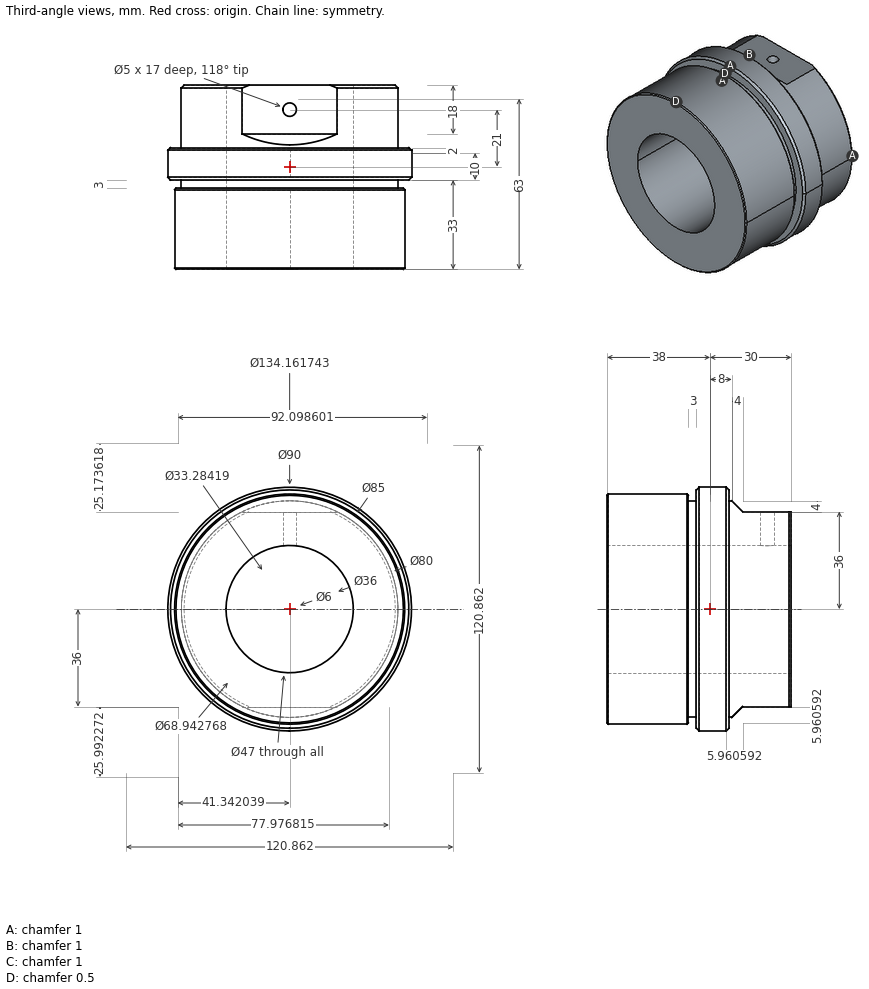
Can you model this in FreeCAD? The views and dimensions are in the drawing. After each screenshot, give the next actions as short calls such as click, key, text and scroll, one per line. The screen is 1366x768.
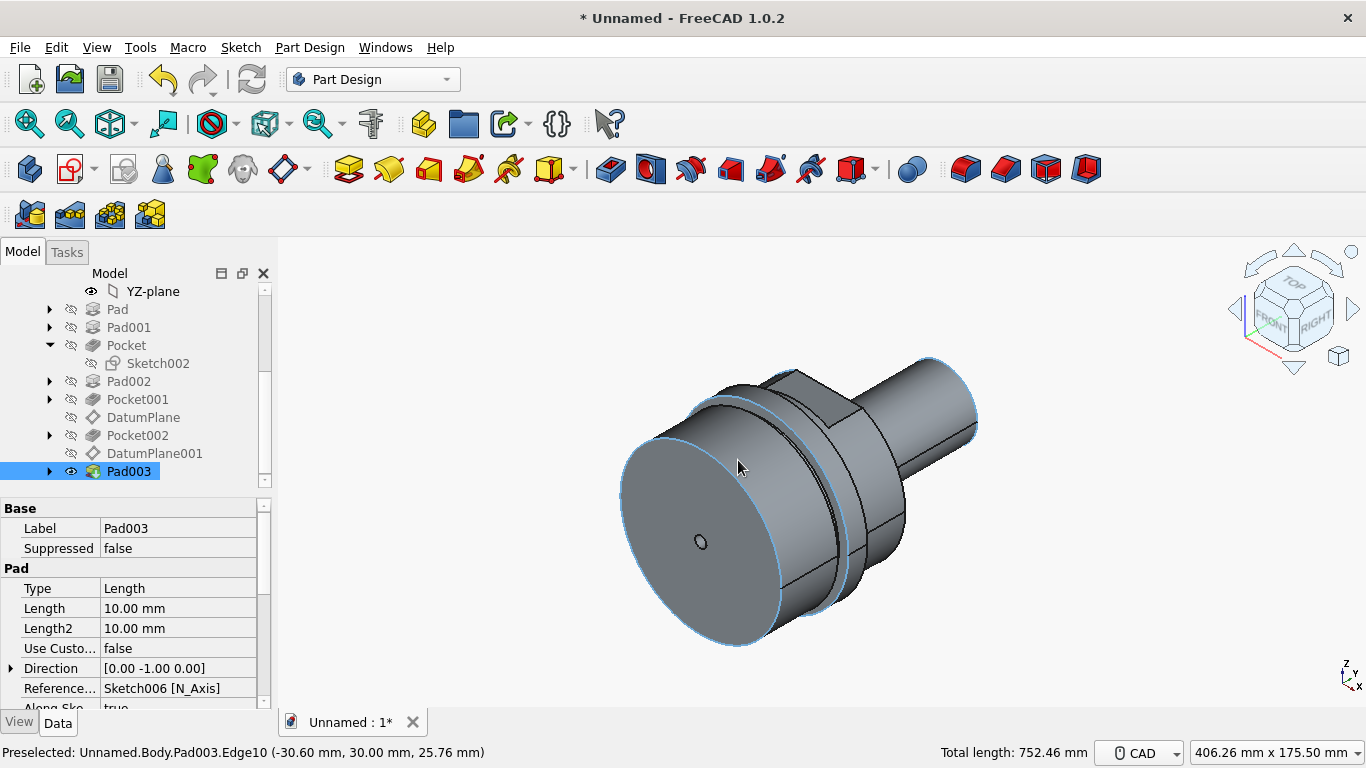
key(1)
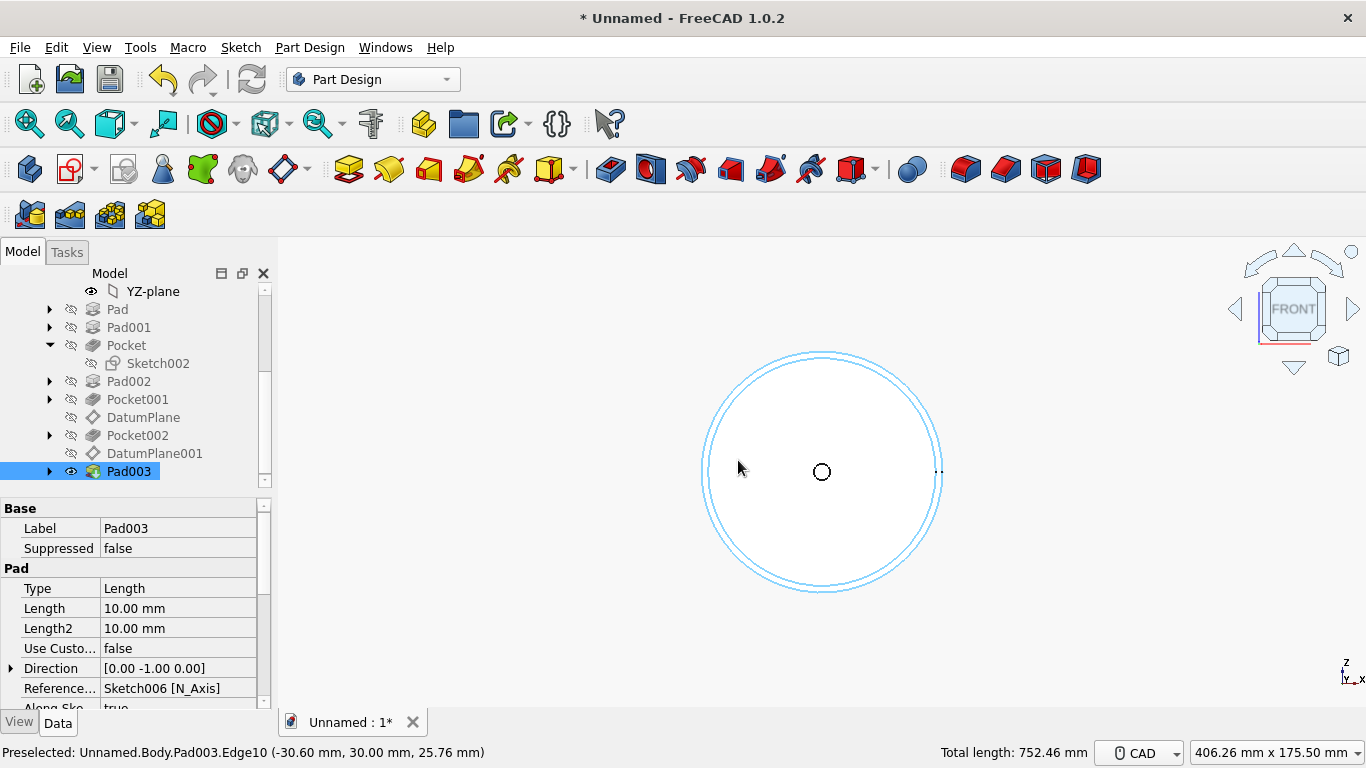
key(3)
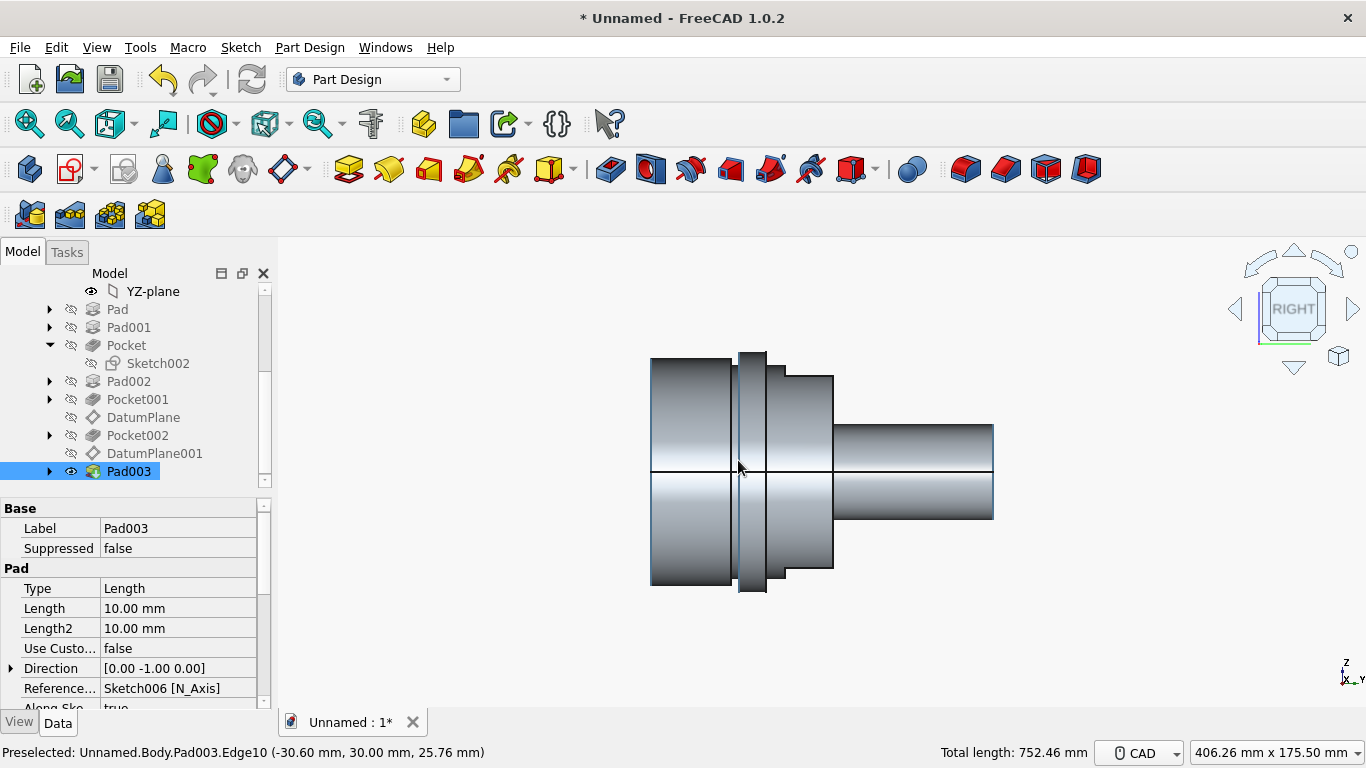
click(833, 517, ctrl)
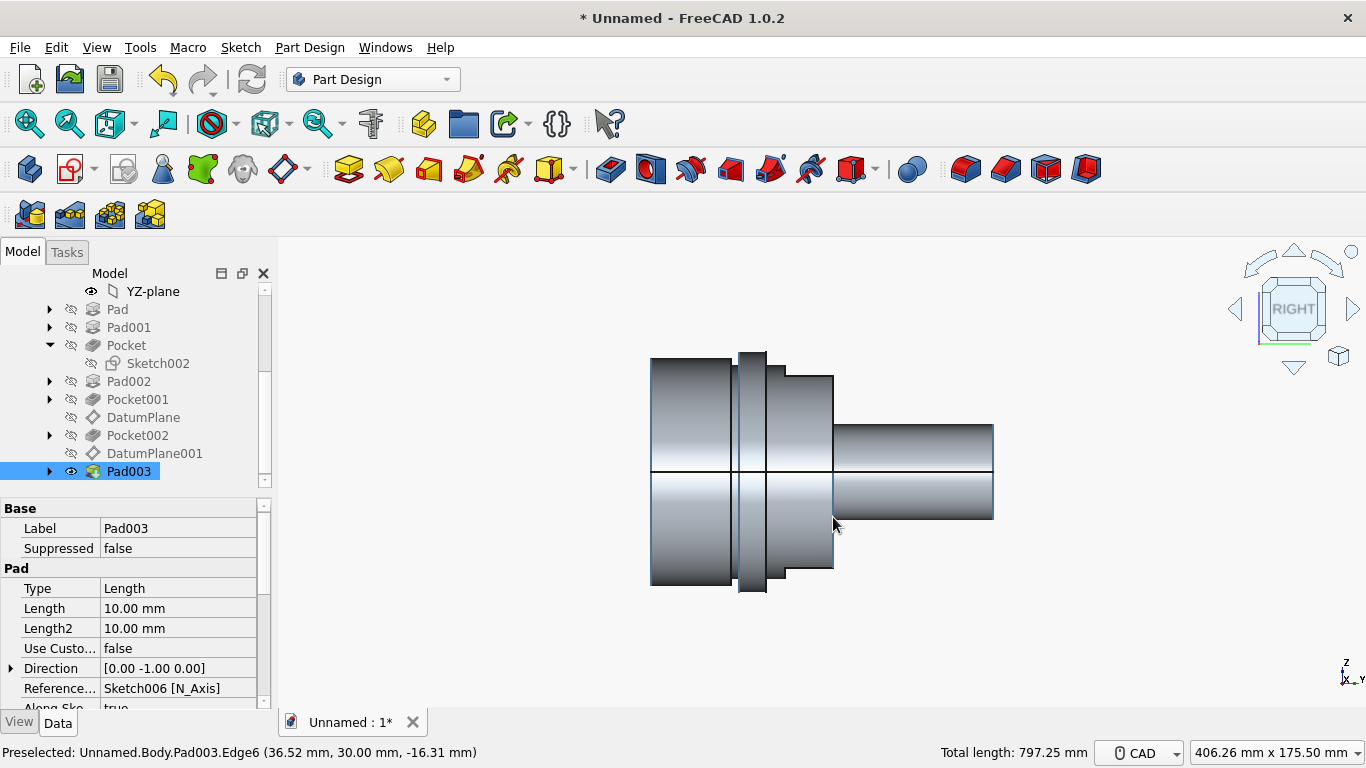
click(1006, 170)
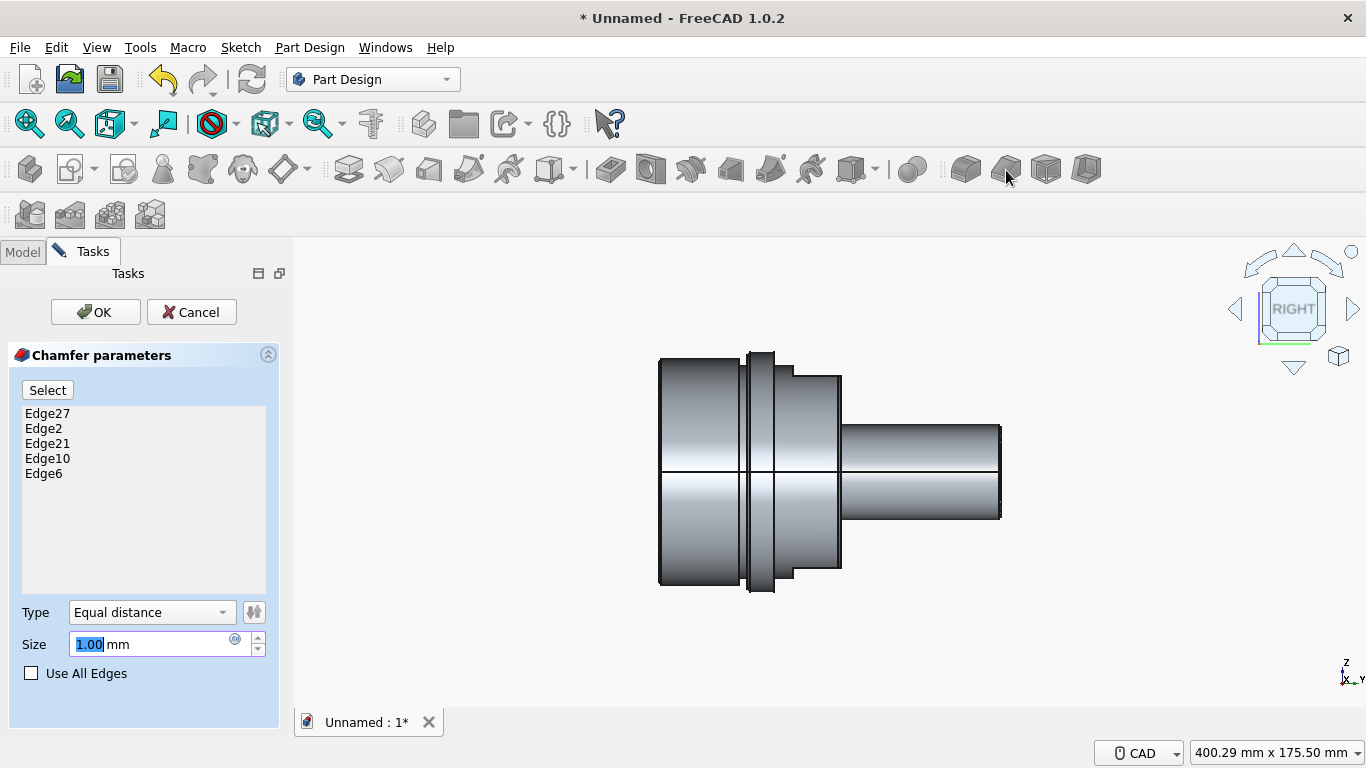
text(1)
key(Tab)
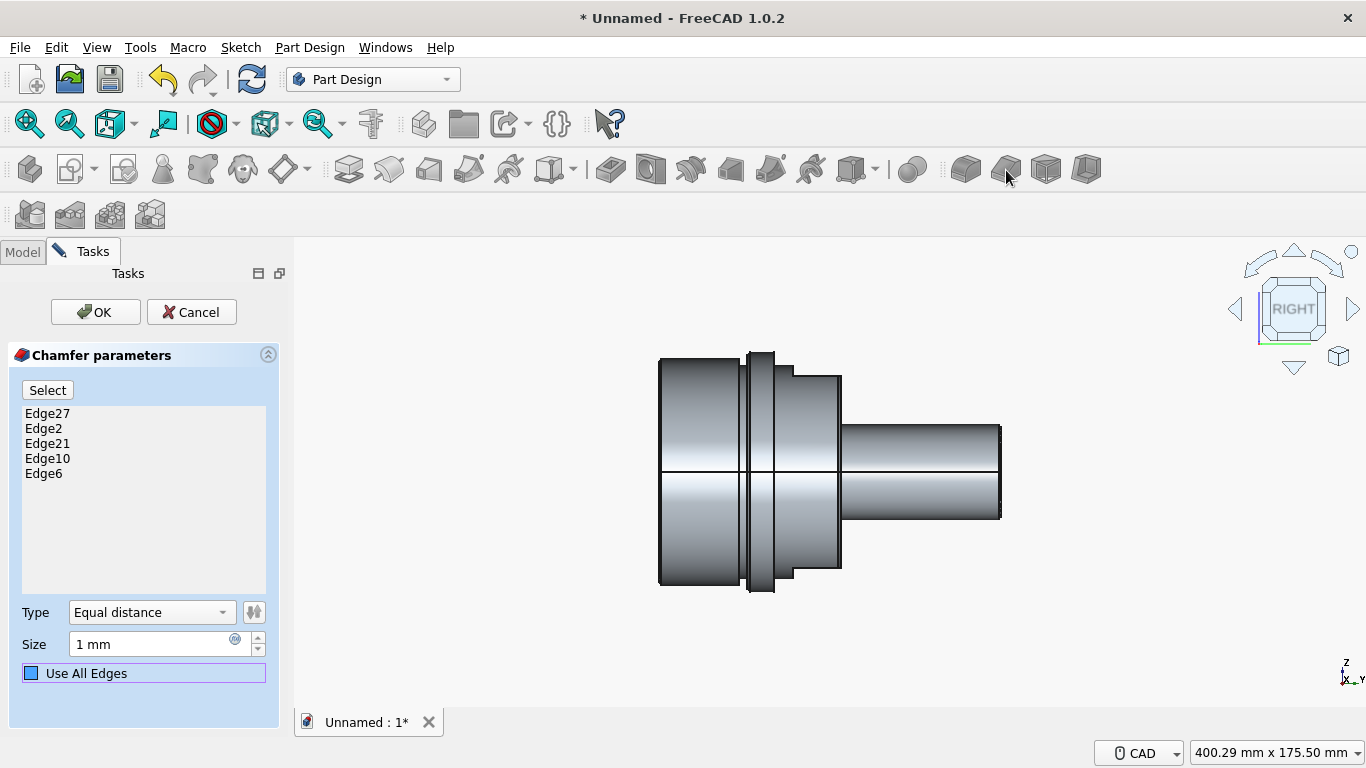
click(96, 312)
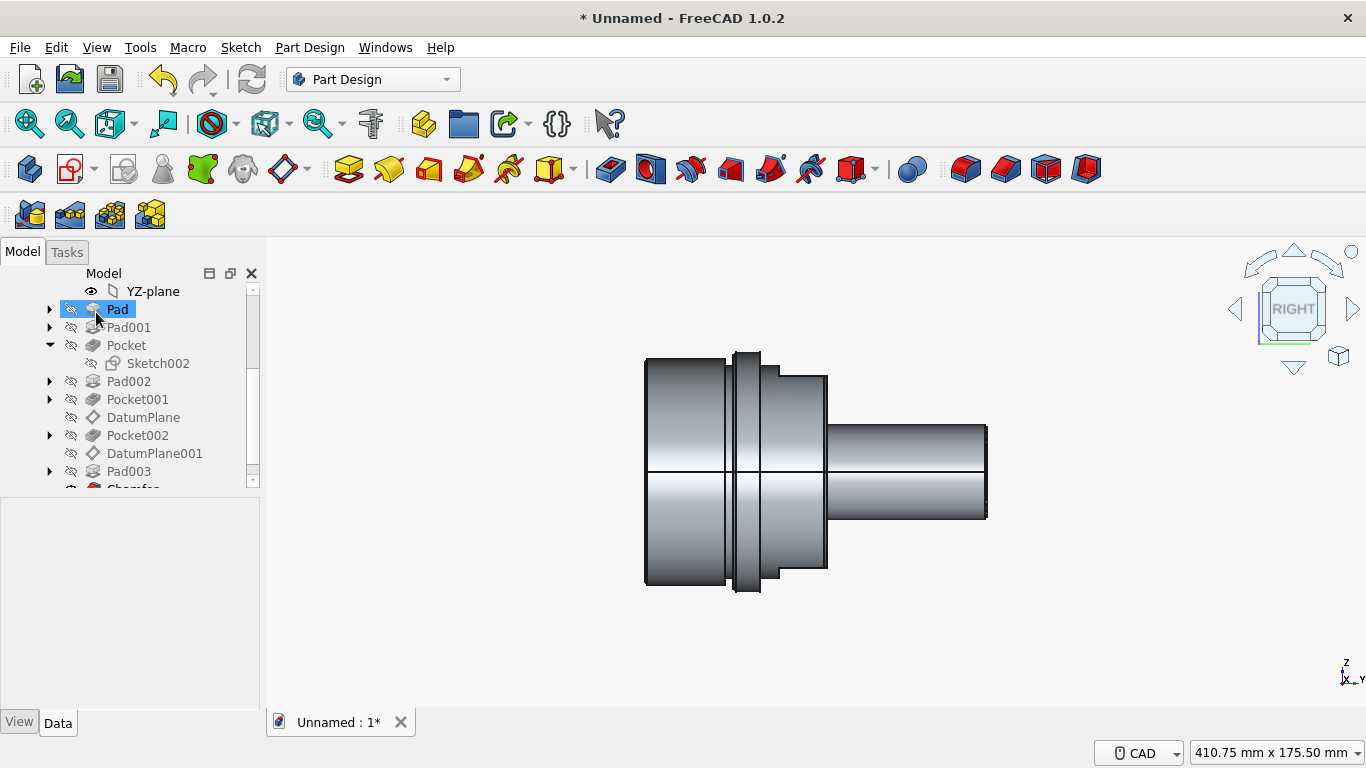
click(70, 170)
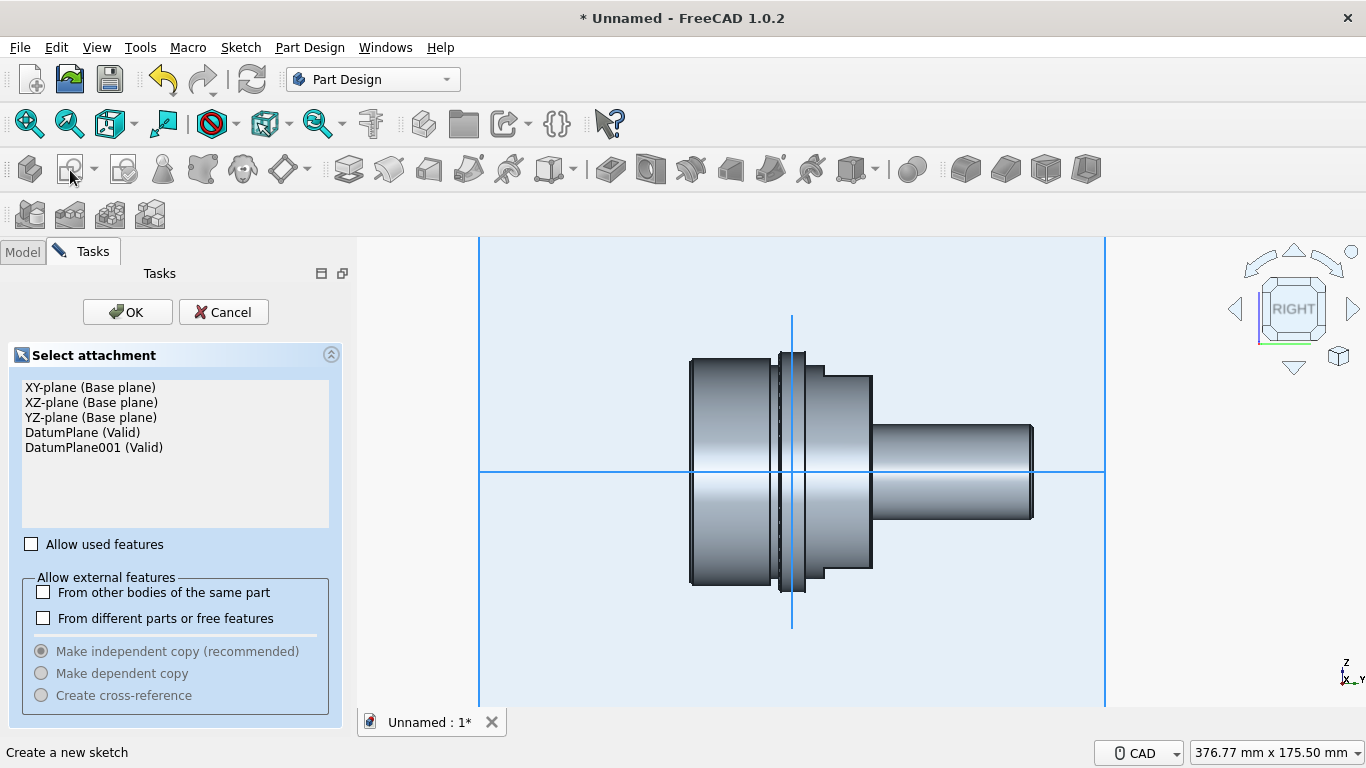
click(82, 418)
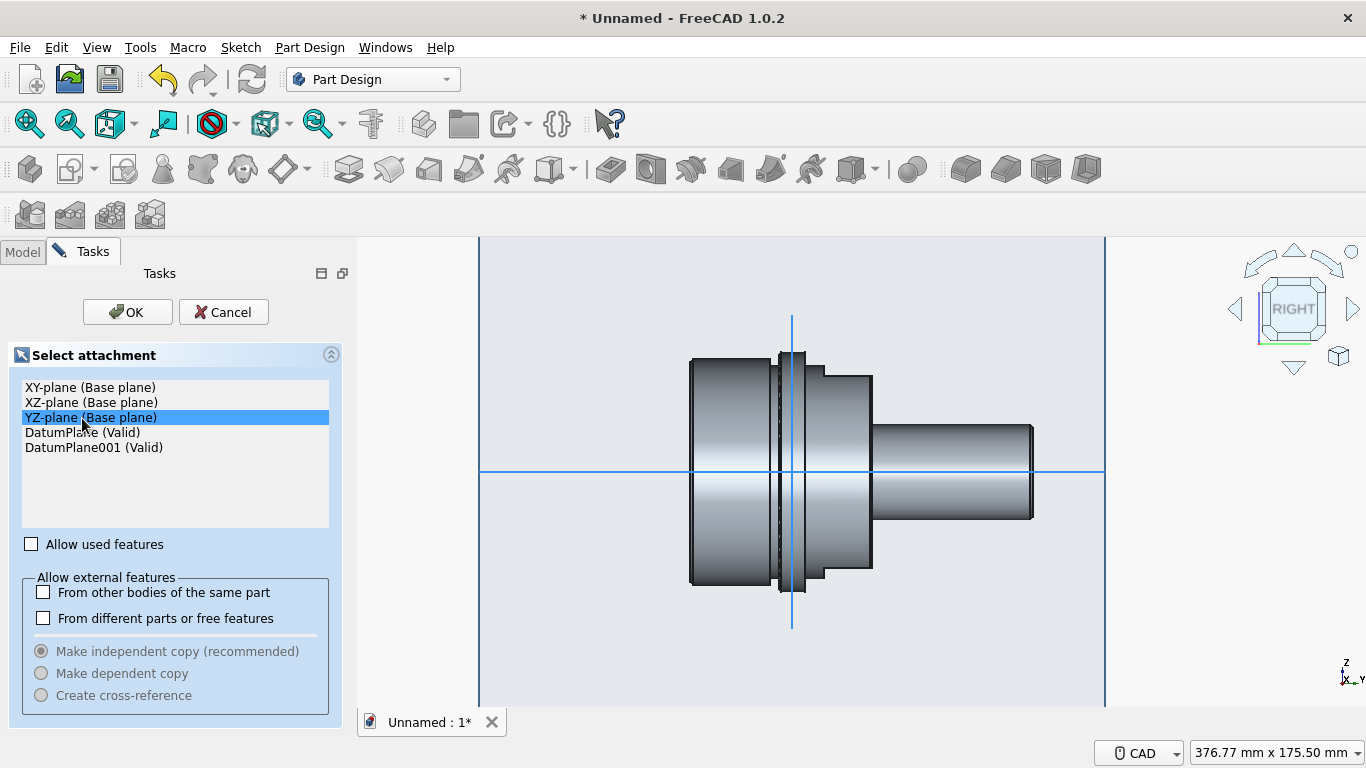
click(128, 312)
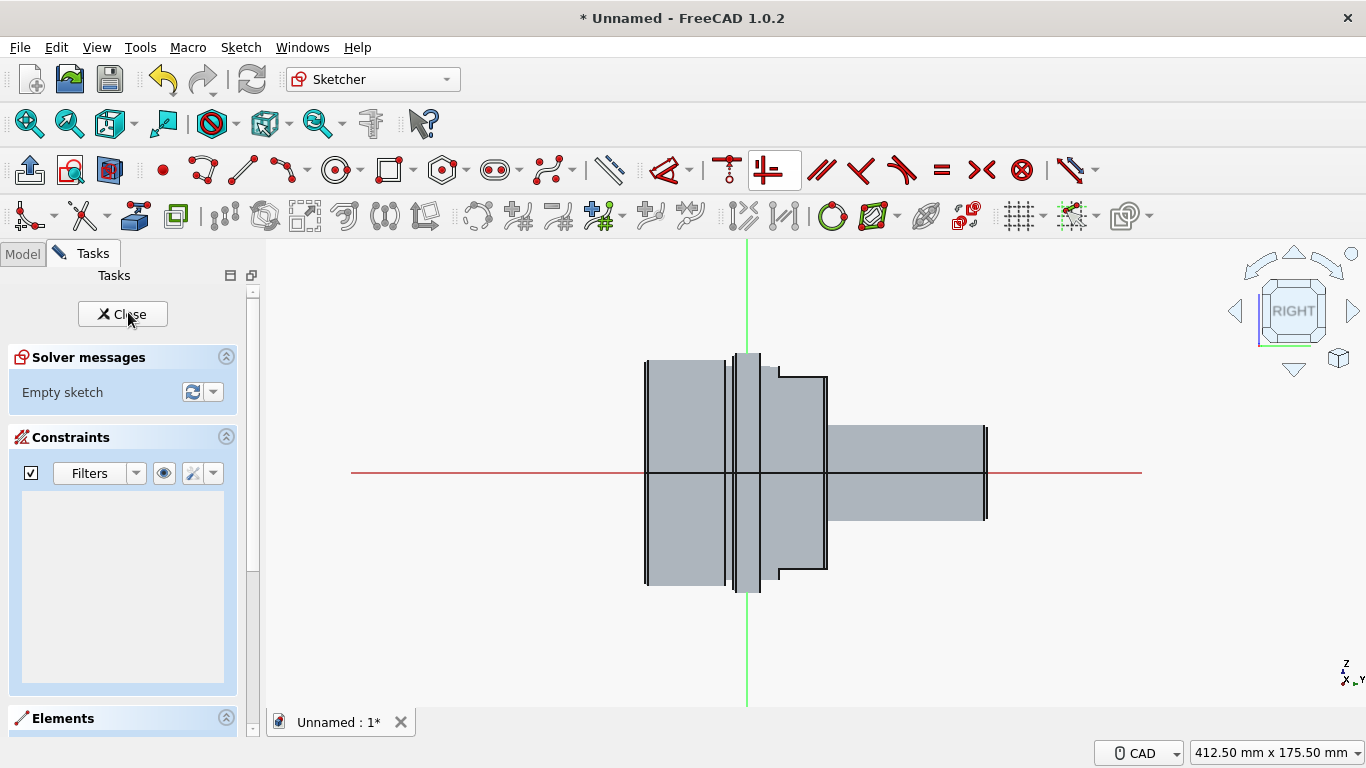
click(110, 170)